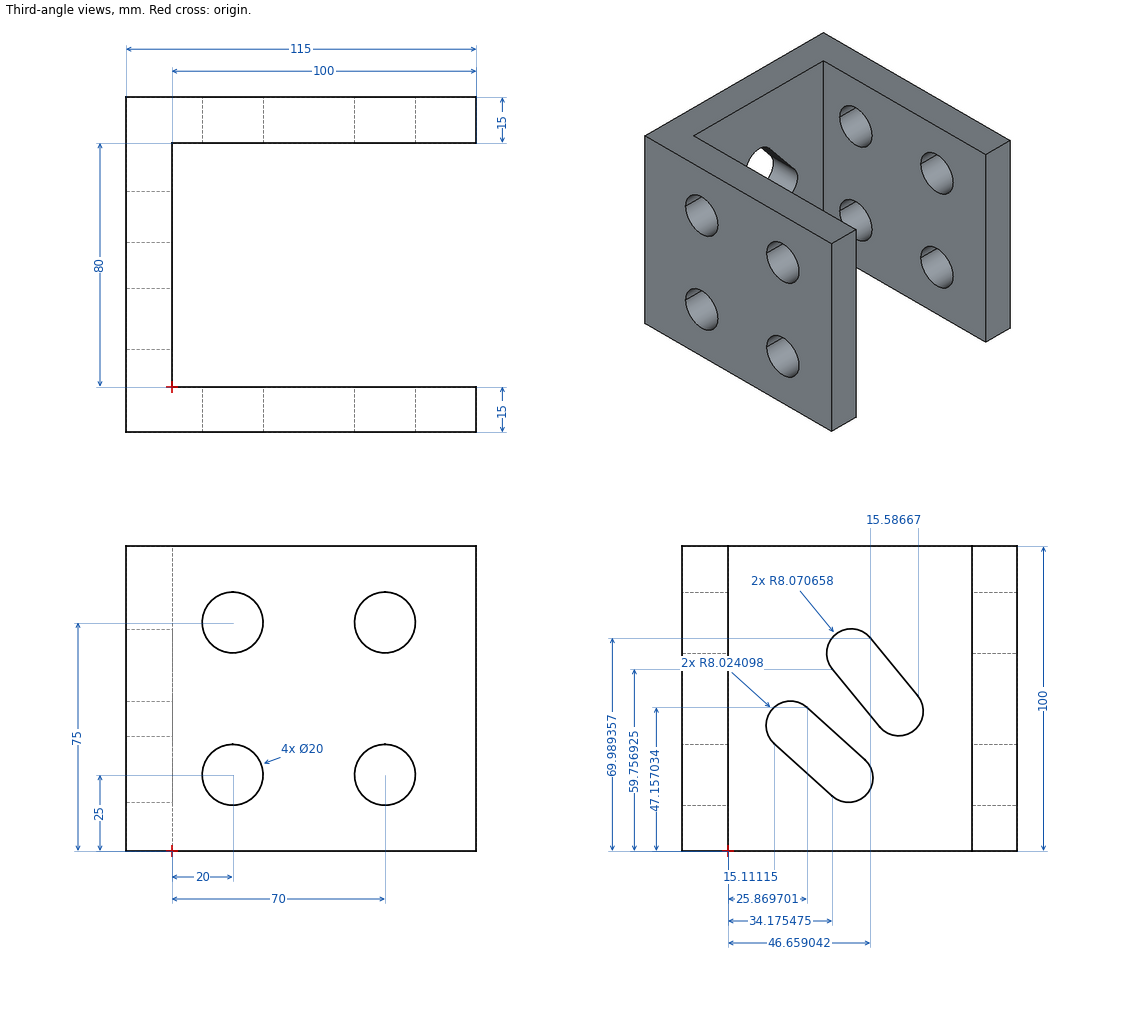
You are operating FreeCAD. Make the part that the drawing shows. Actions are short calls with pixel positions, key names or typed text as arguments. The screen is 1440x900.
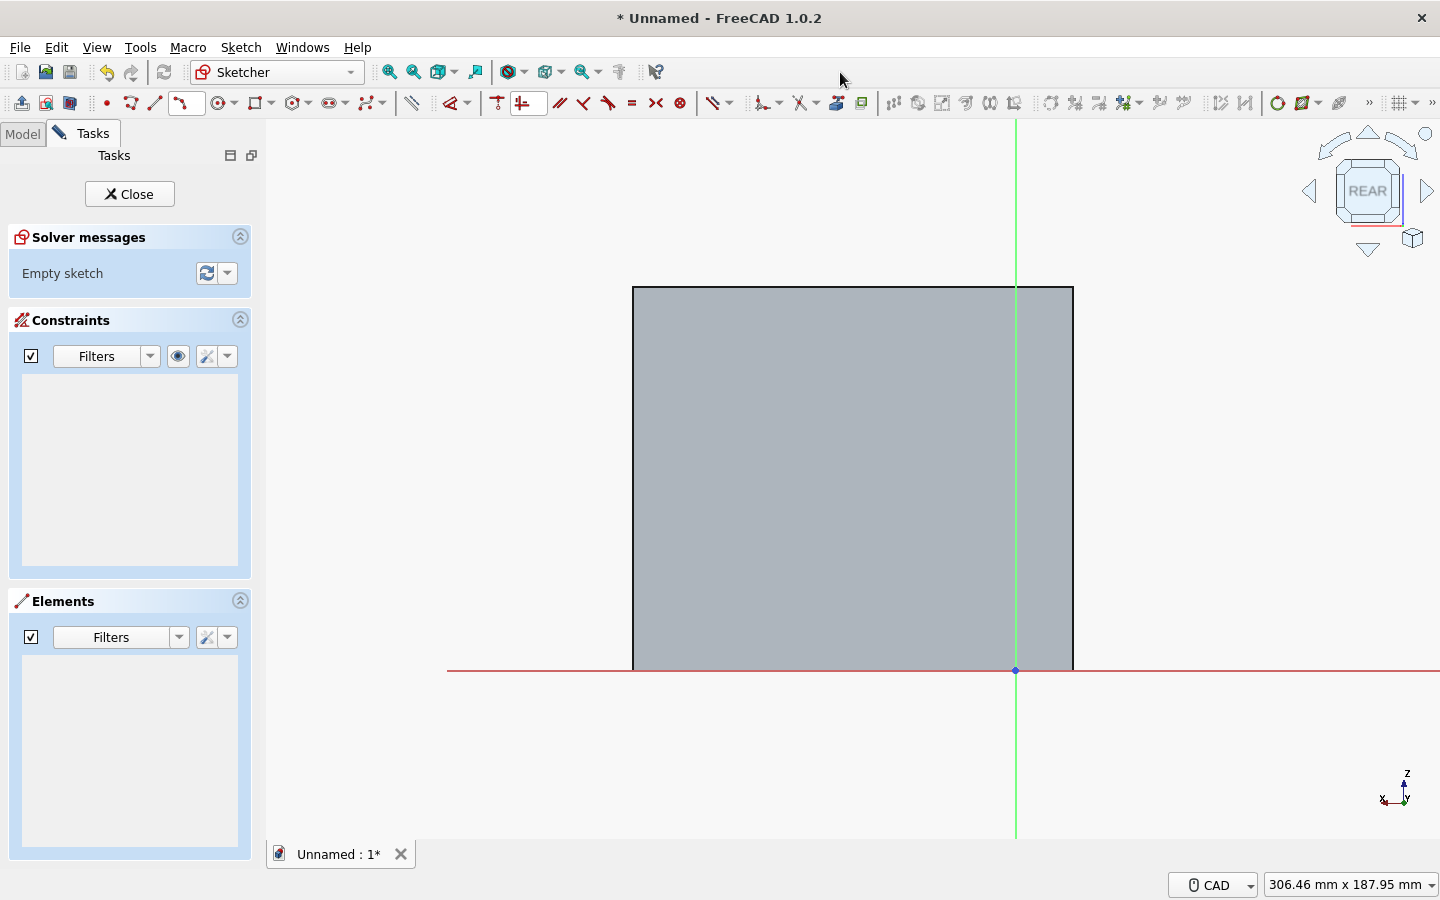
scroll(1021, 566, up, 2)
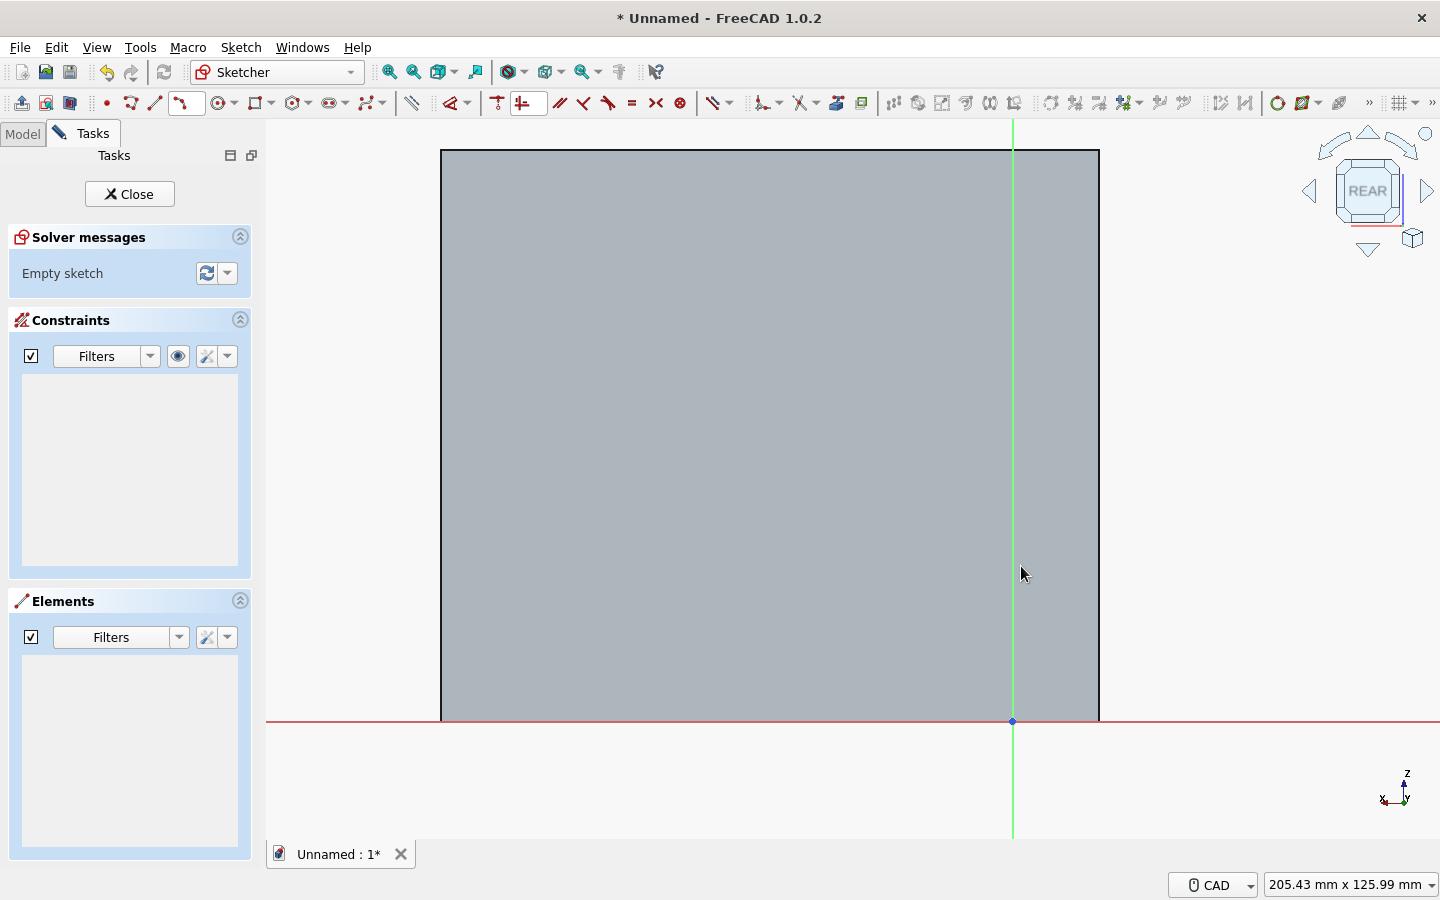
key(g)
key(c)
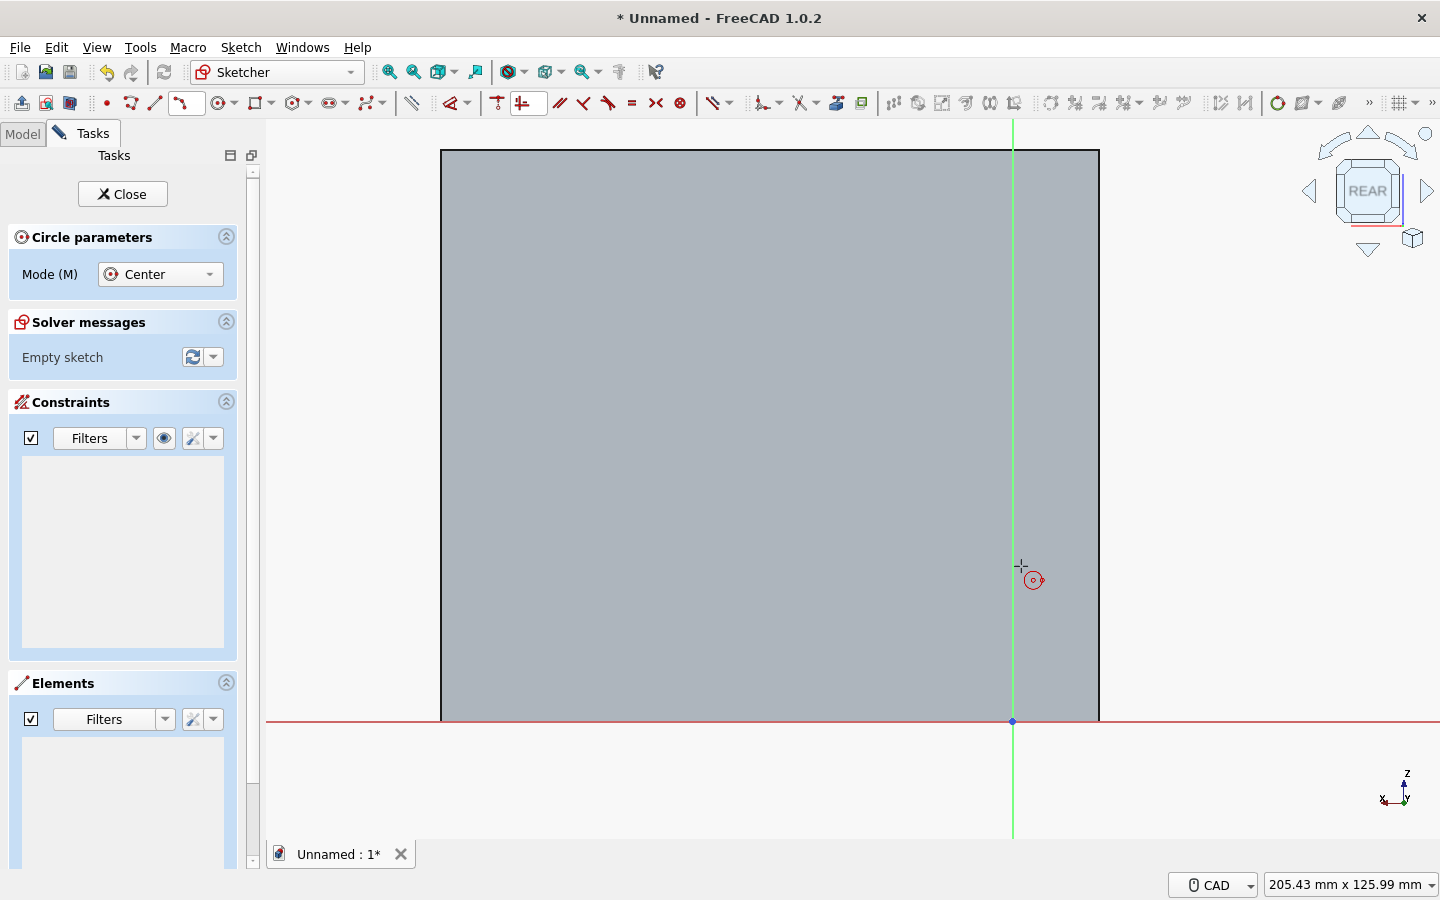
click(899, 579)
move(939, 538)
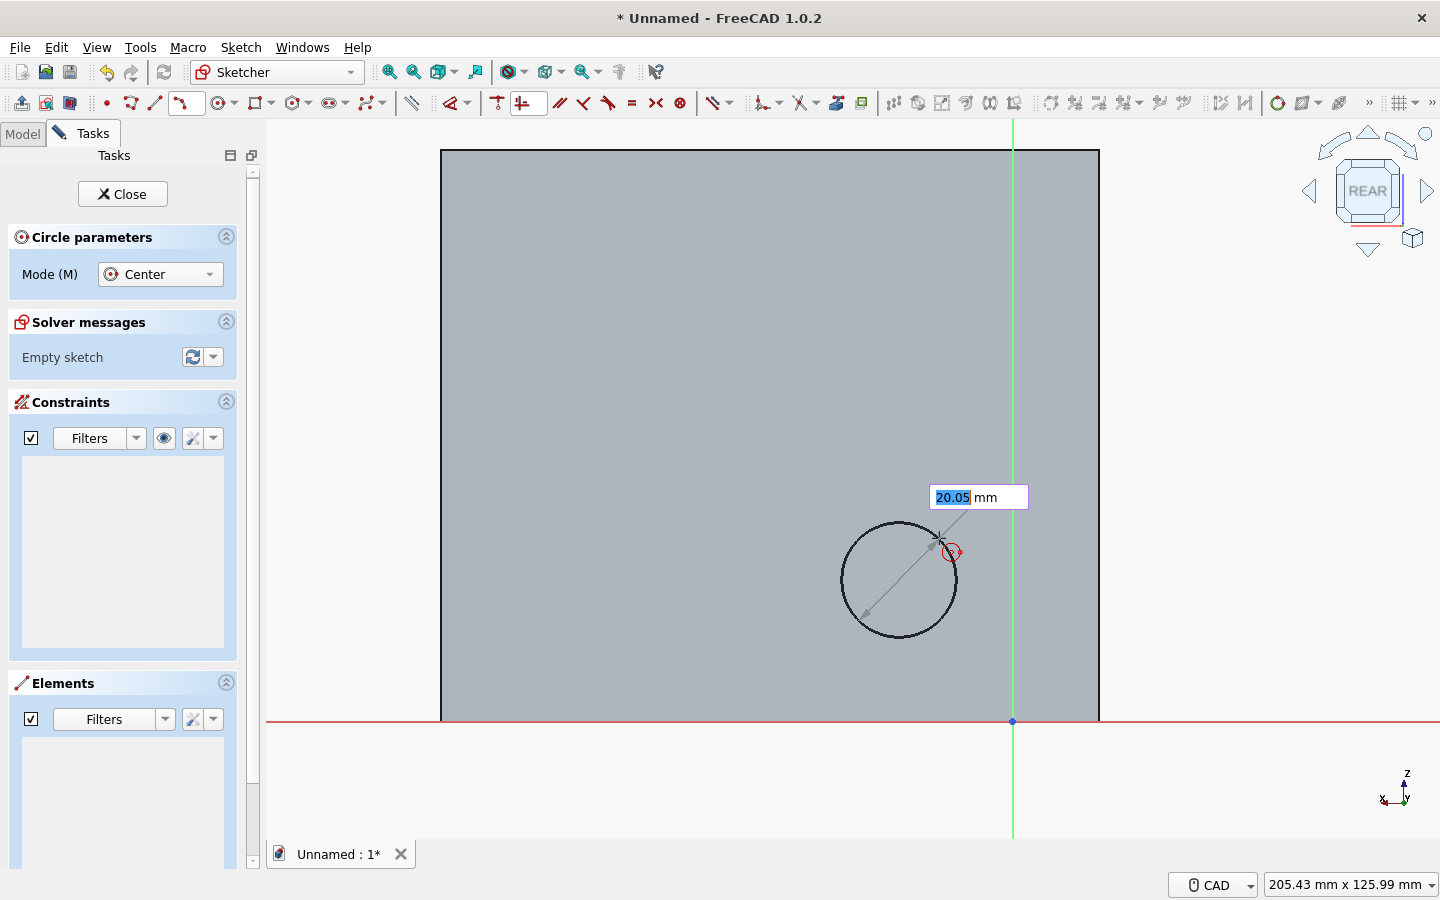
text(20)
key(Return)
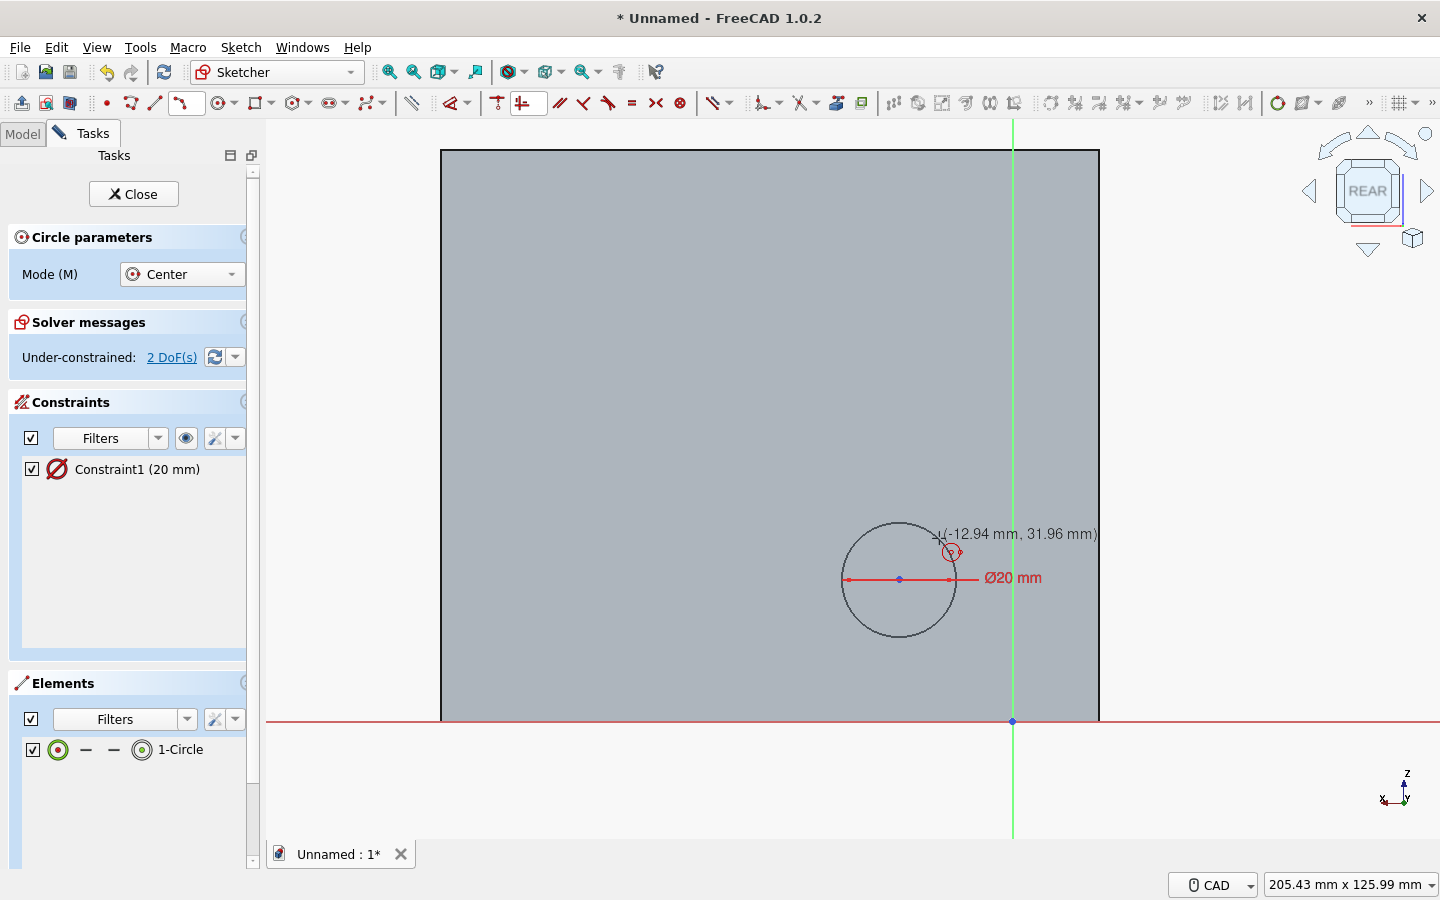
click(613, 579)
move(653, 538)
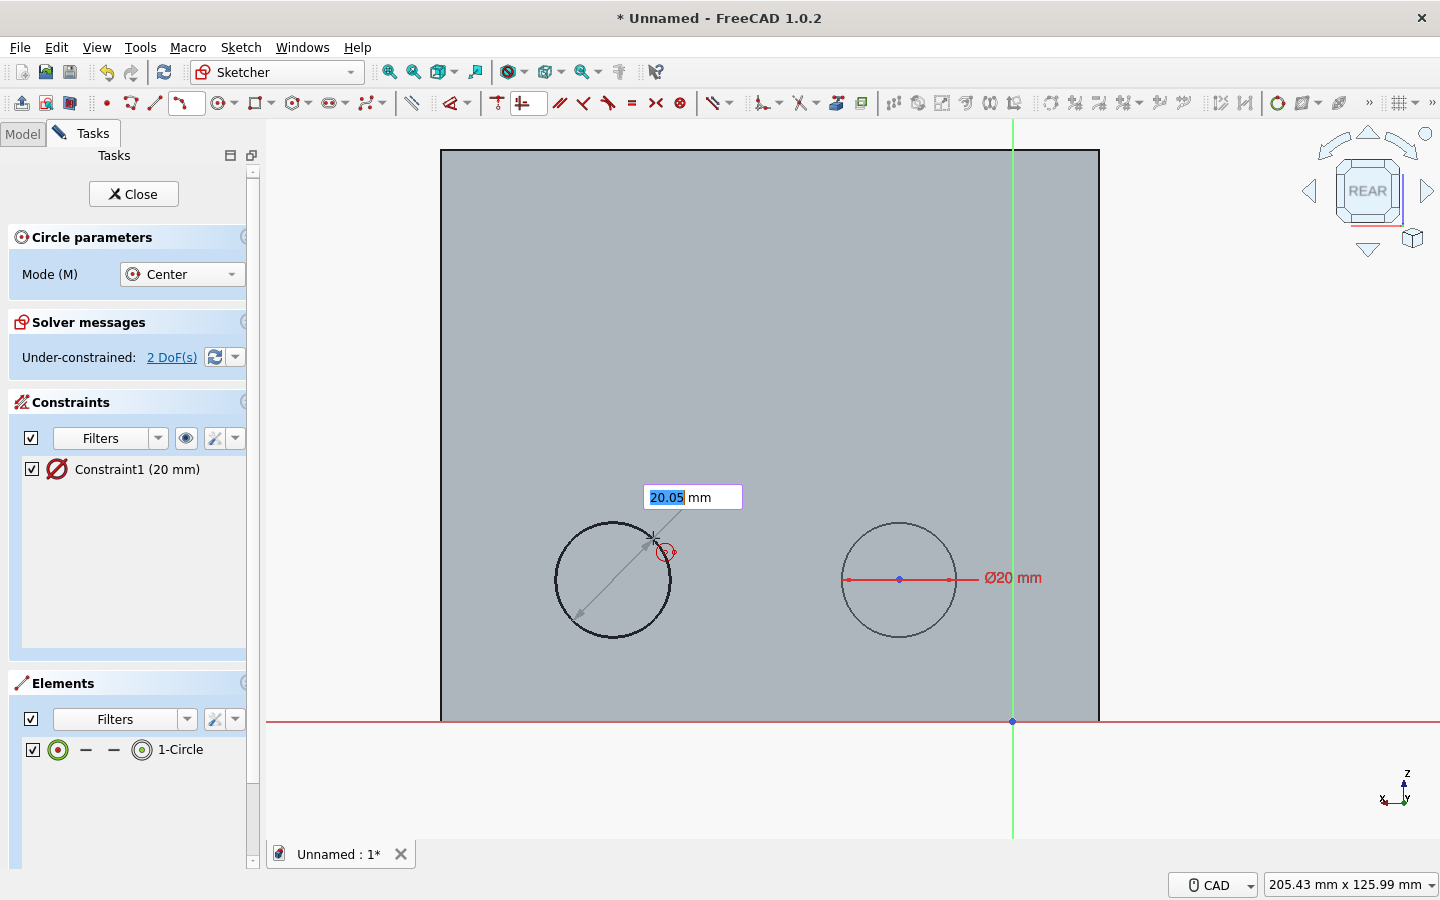
text(20)
key(Return)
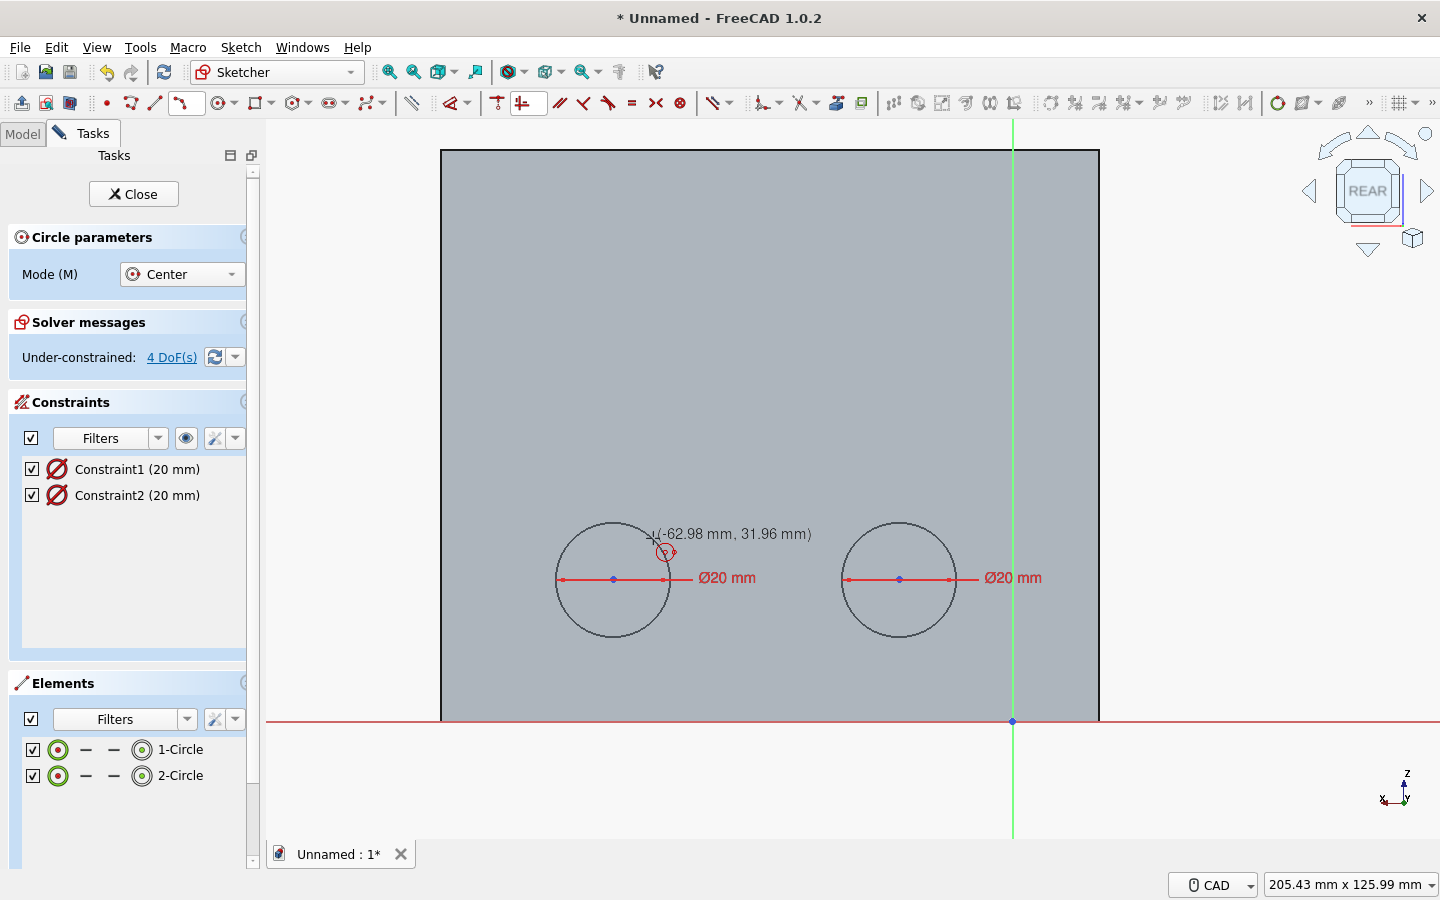
click(899, 293)
move(939, 253)